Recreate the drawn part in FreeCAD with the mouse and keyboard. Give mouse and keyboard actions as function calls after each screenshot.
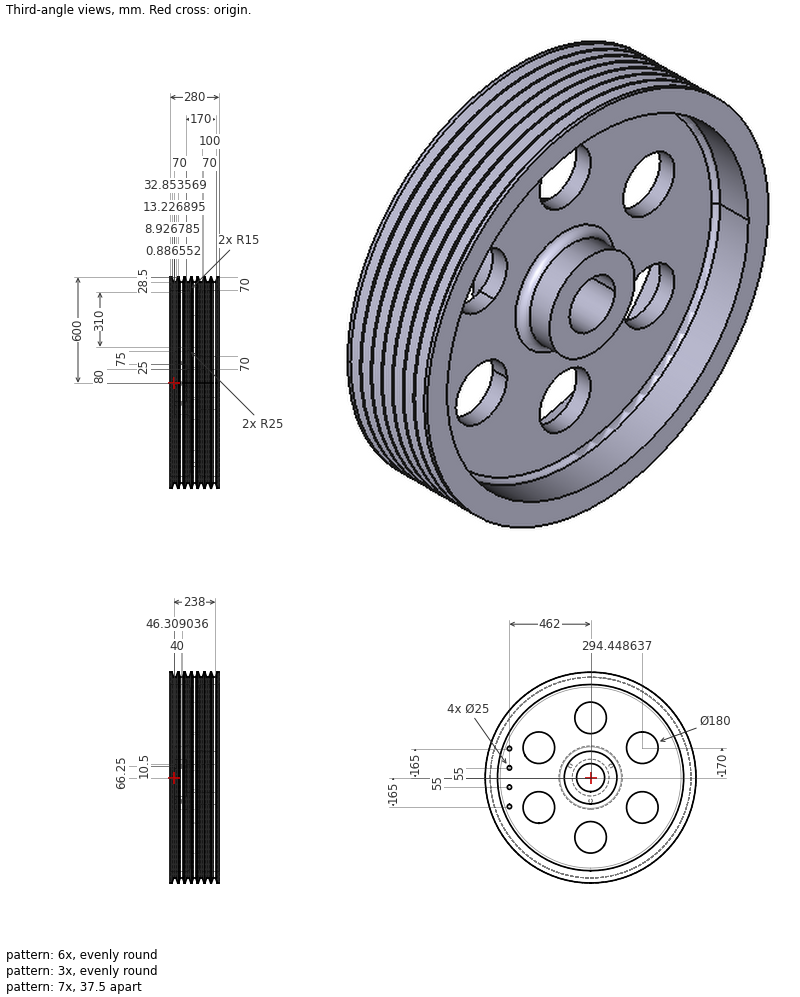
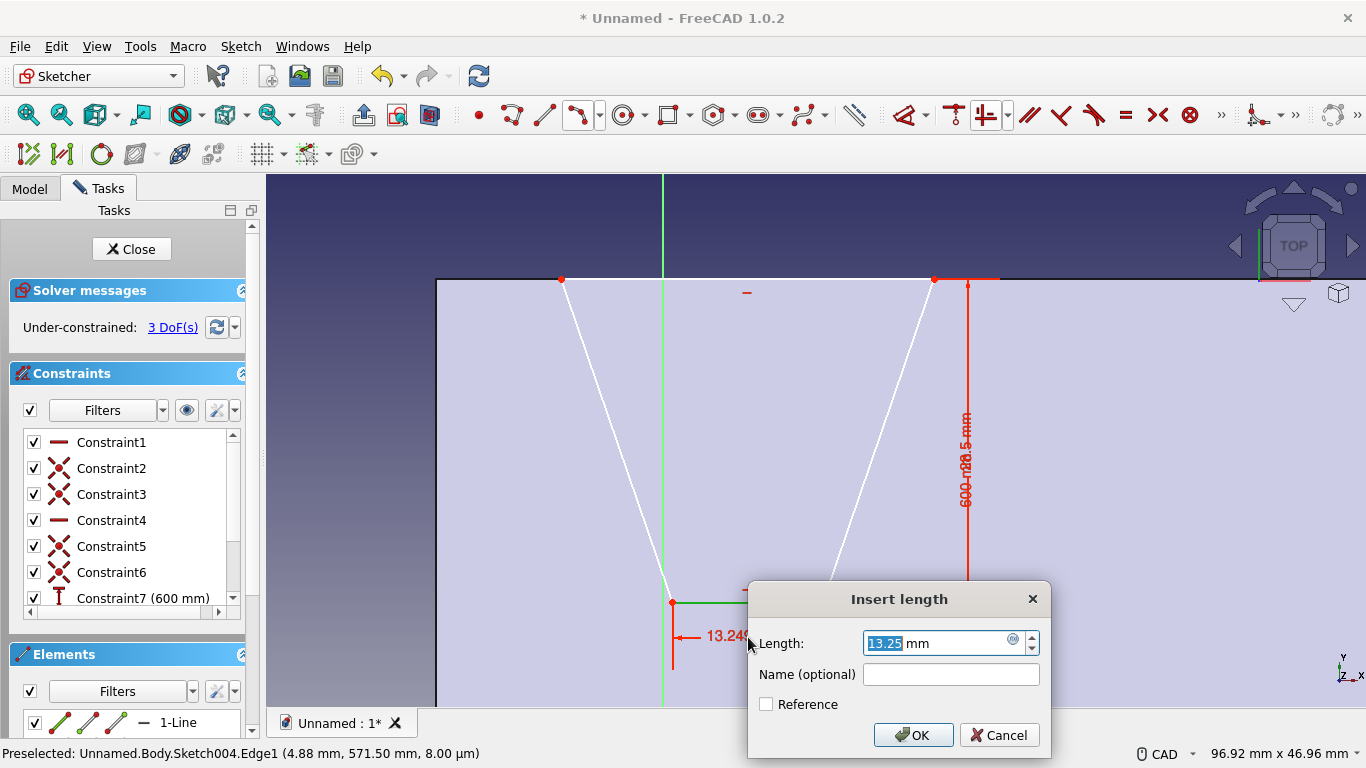
text(13.226895)
key(Return)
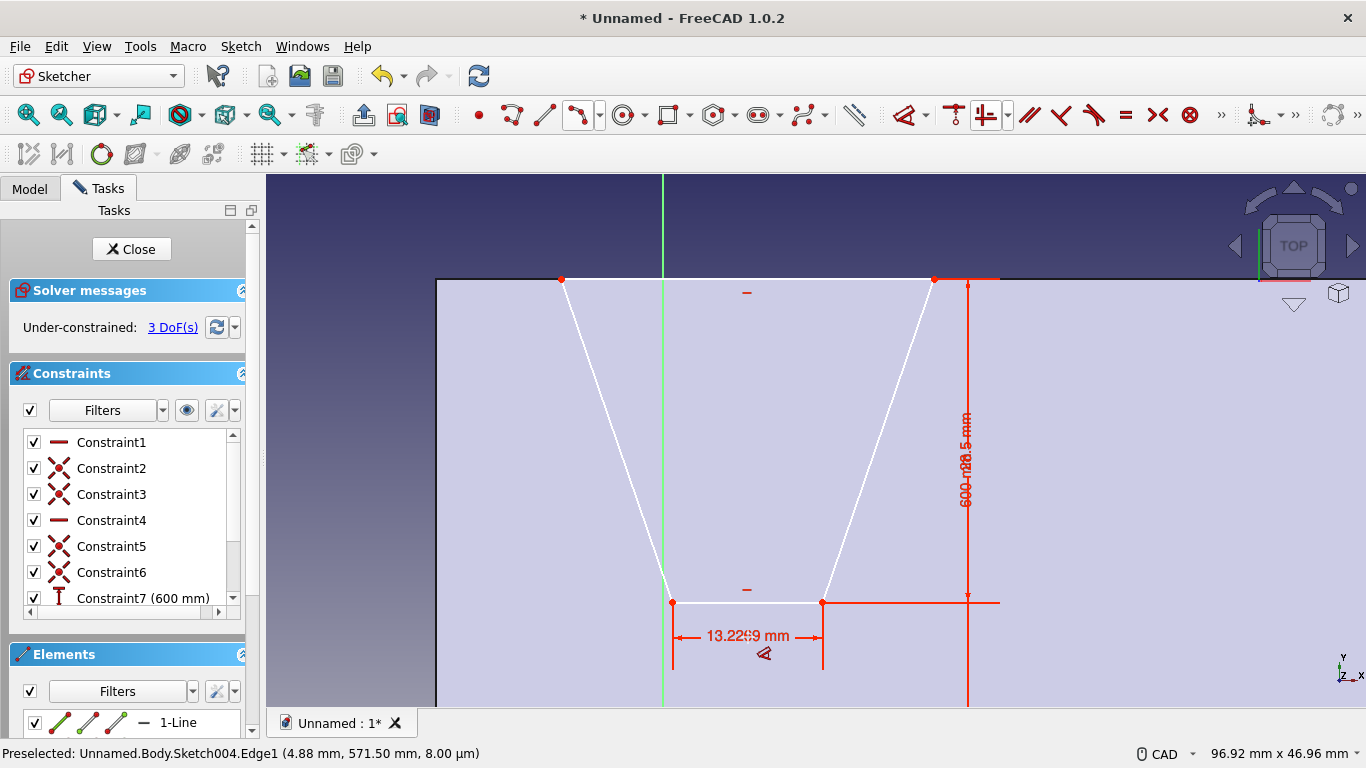
click(822, 279)
click(748, 245)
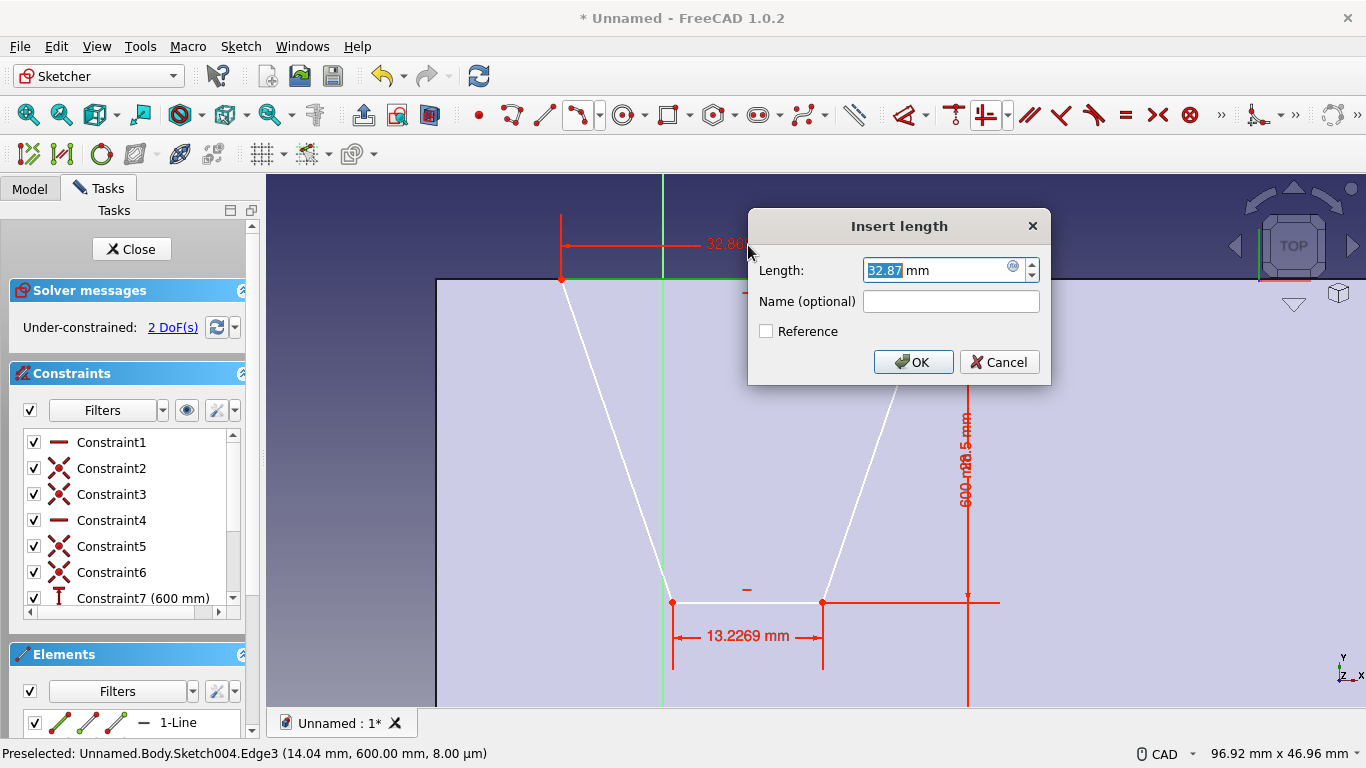
text(32.853569)
key(Return)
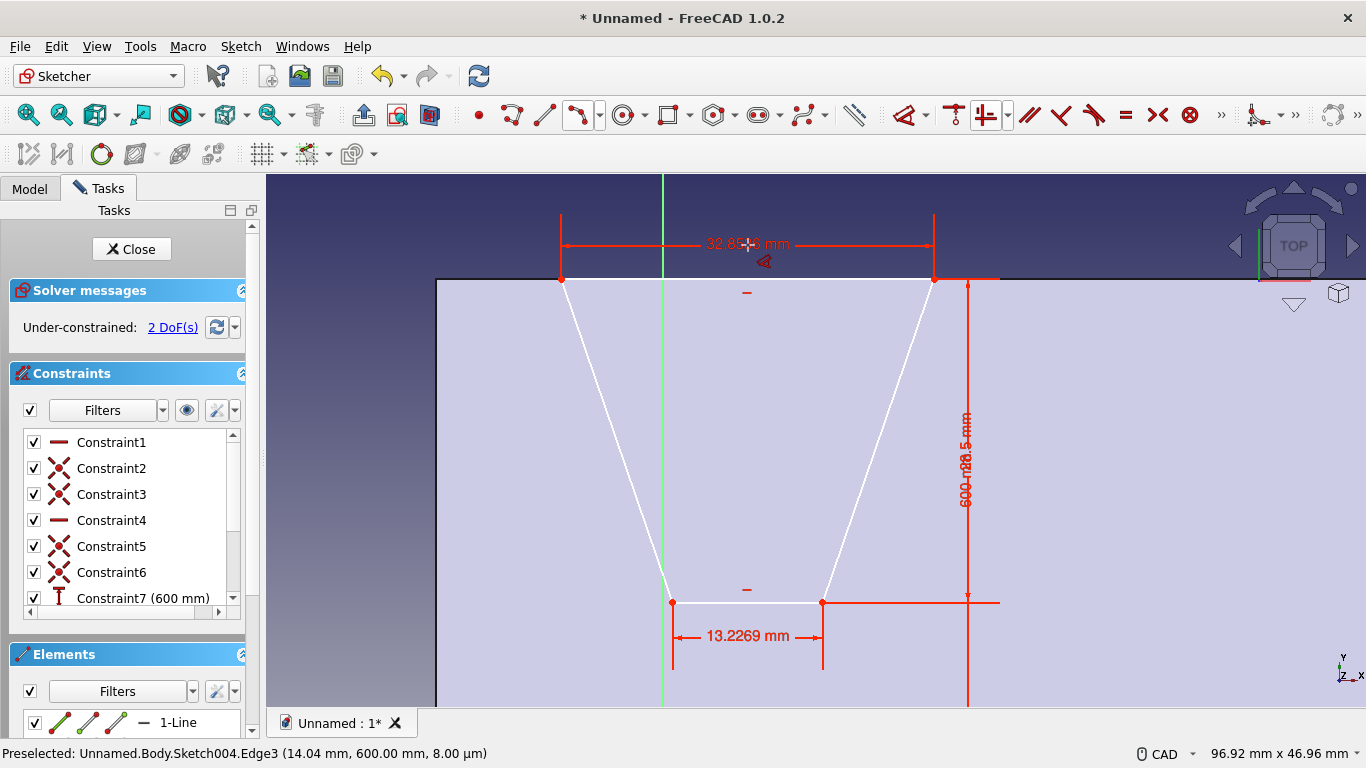
scroll(673, 603, up, 7)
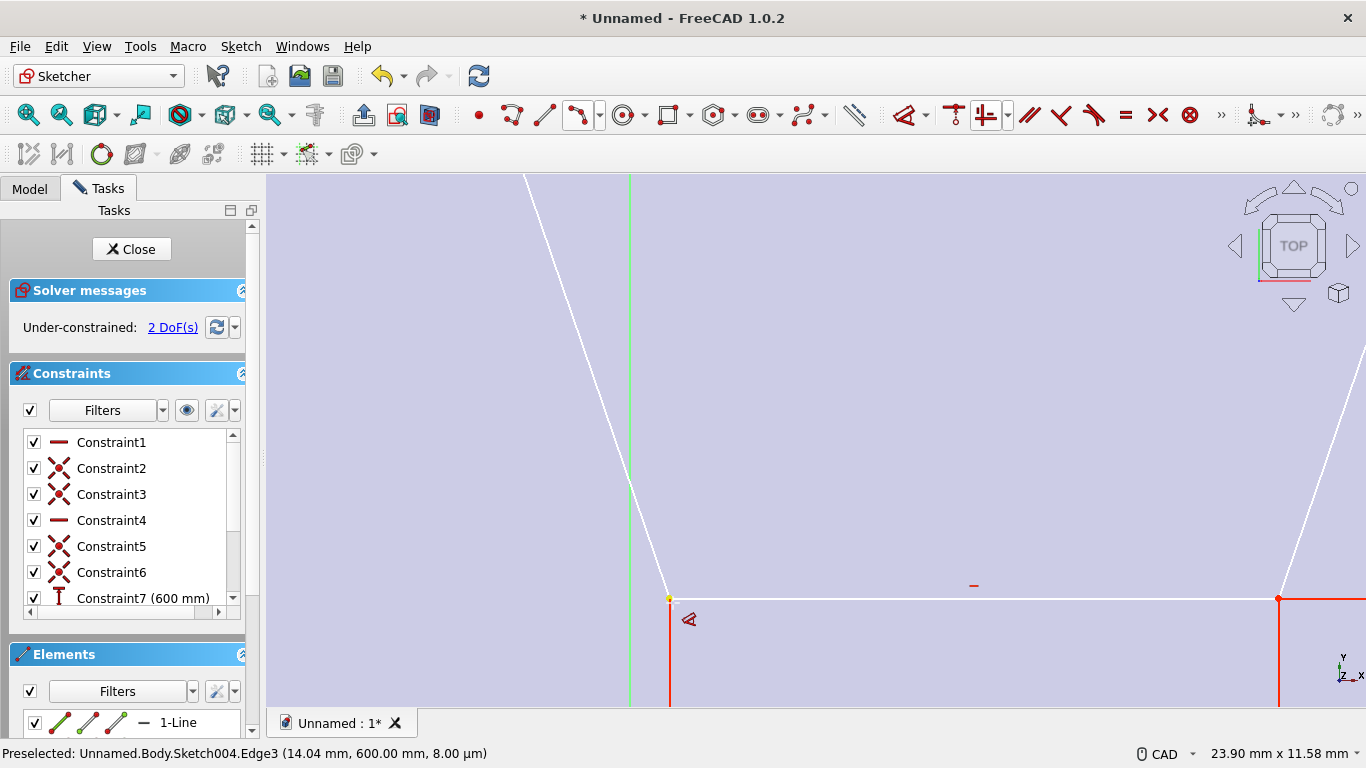
click(670, 599)
click(664, 541)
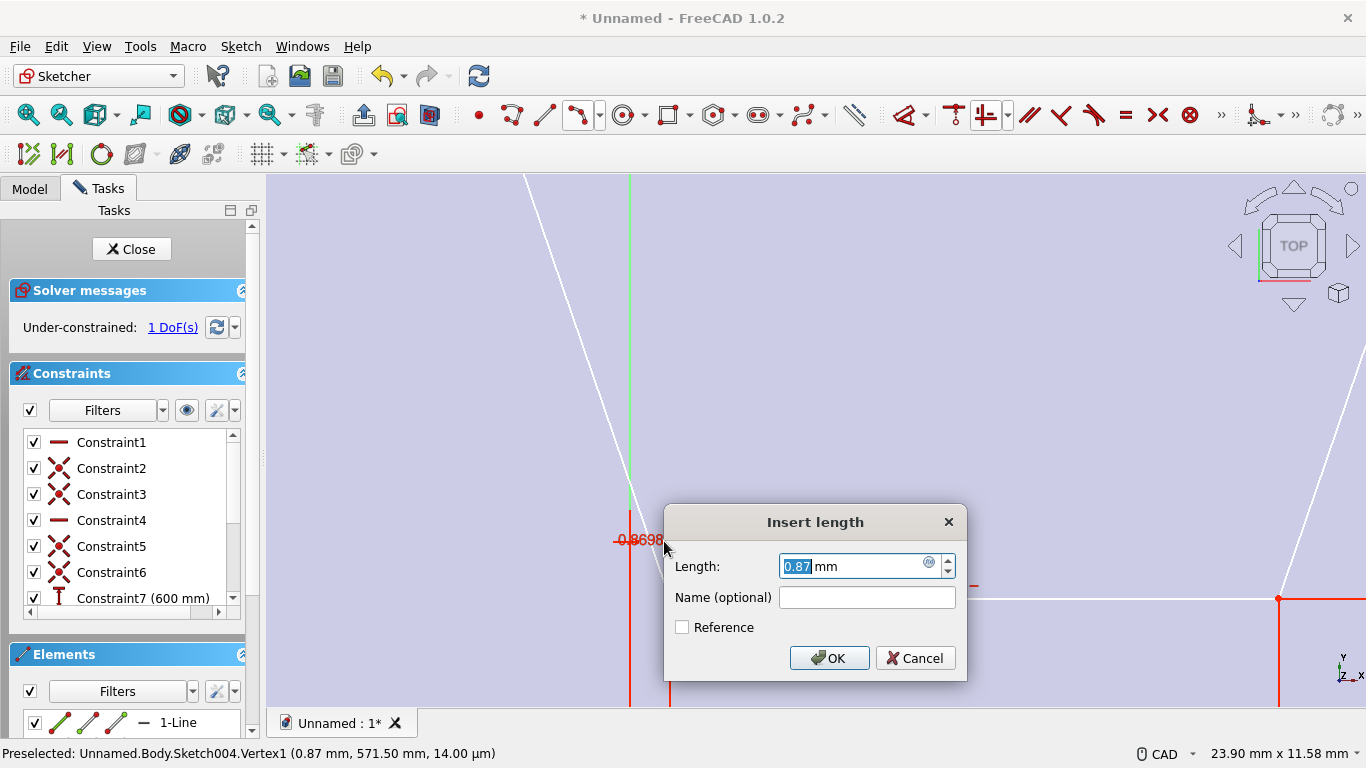
text(0.886552)
key(Return)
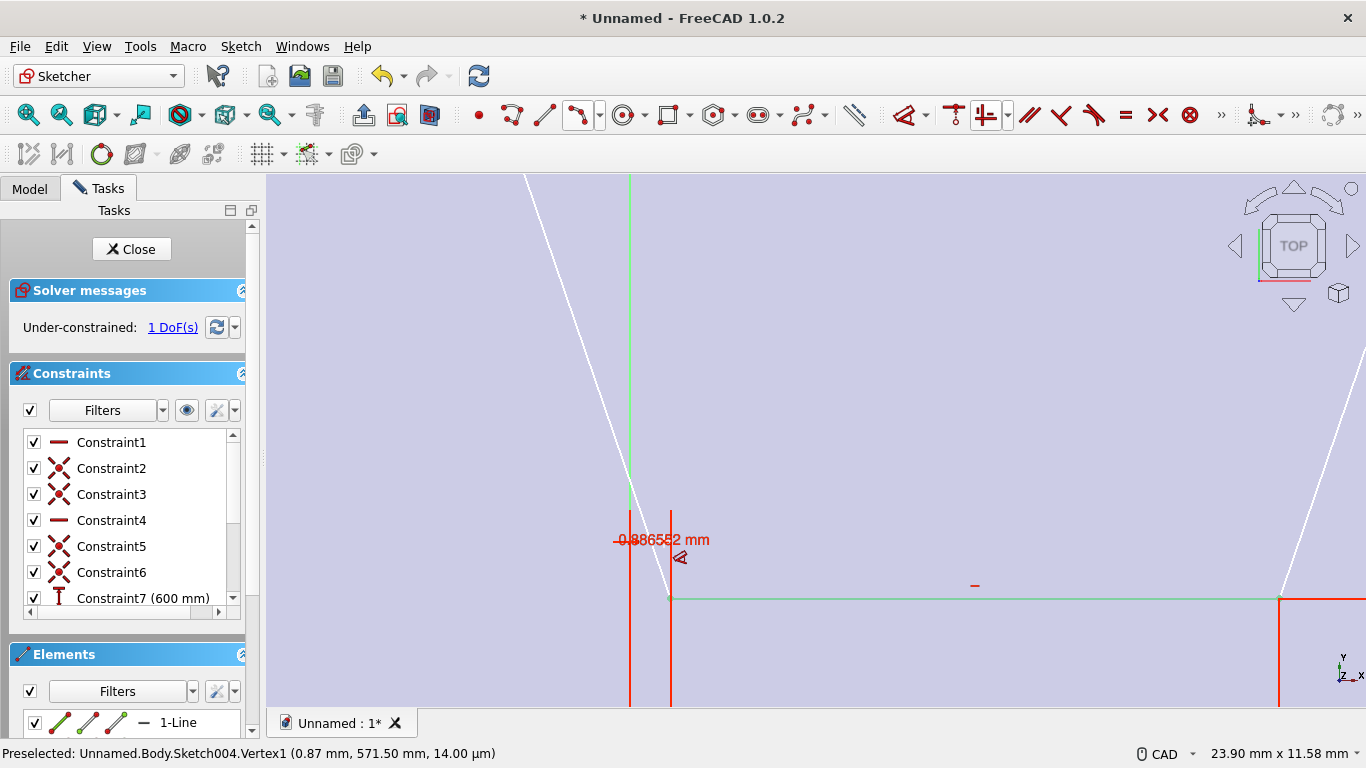
scroll(673, 603, down, 7)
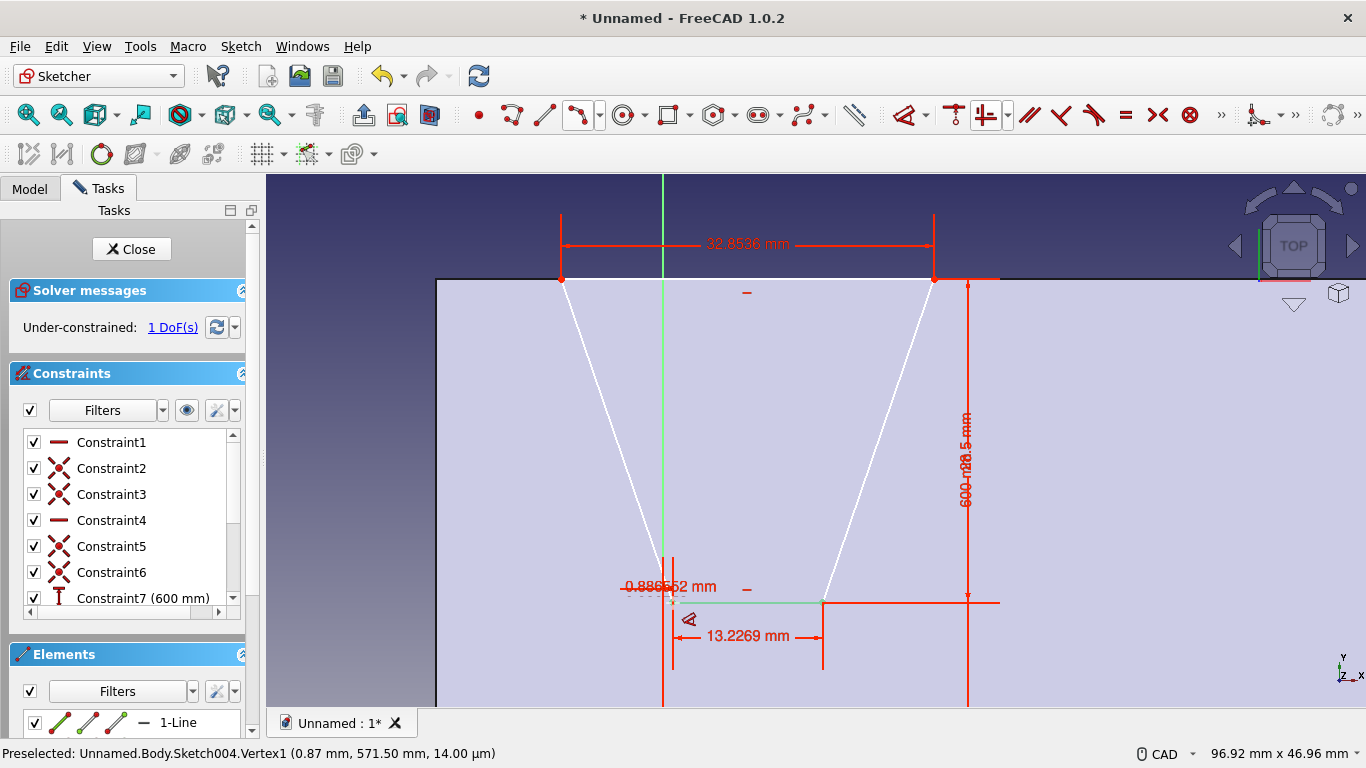
click(561, 279)
click(612, 245)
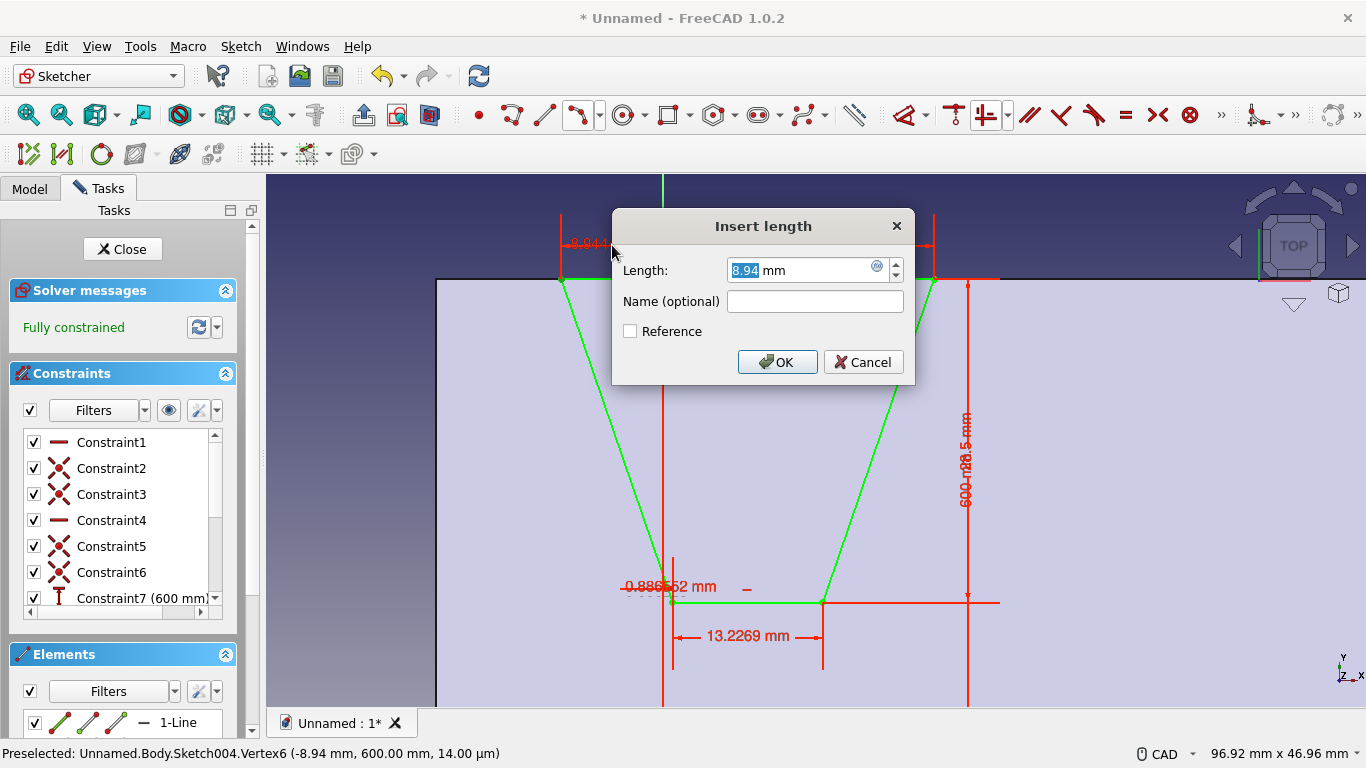
text(8.926785)
key(Return)
key(Escape)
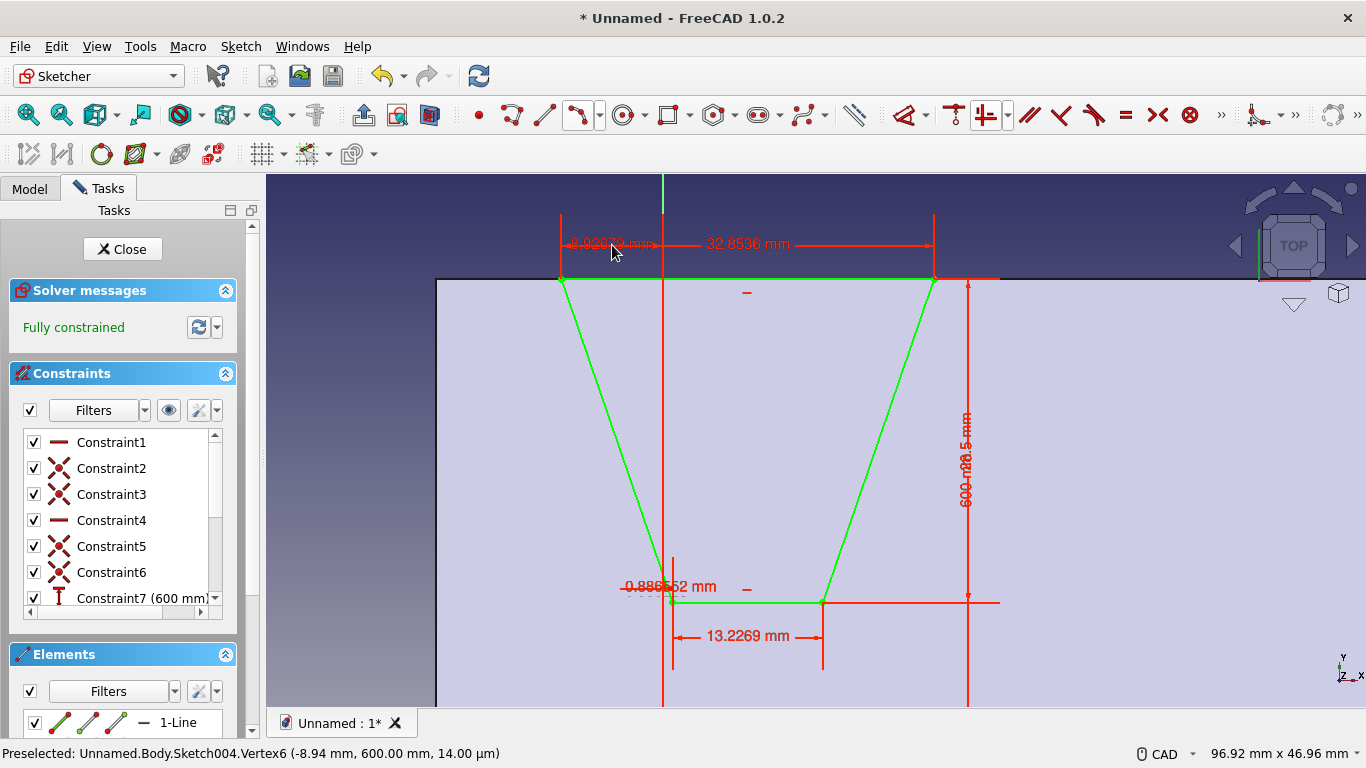
click(123, 249)